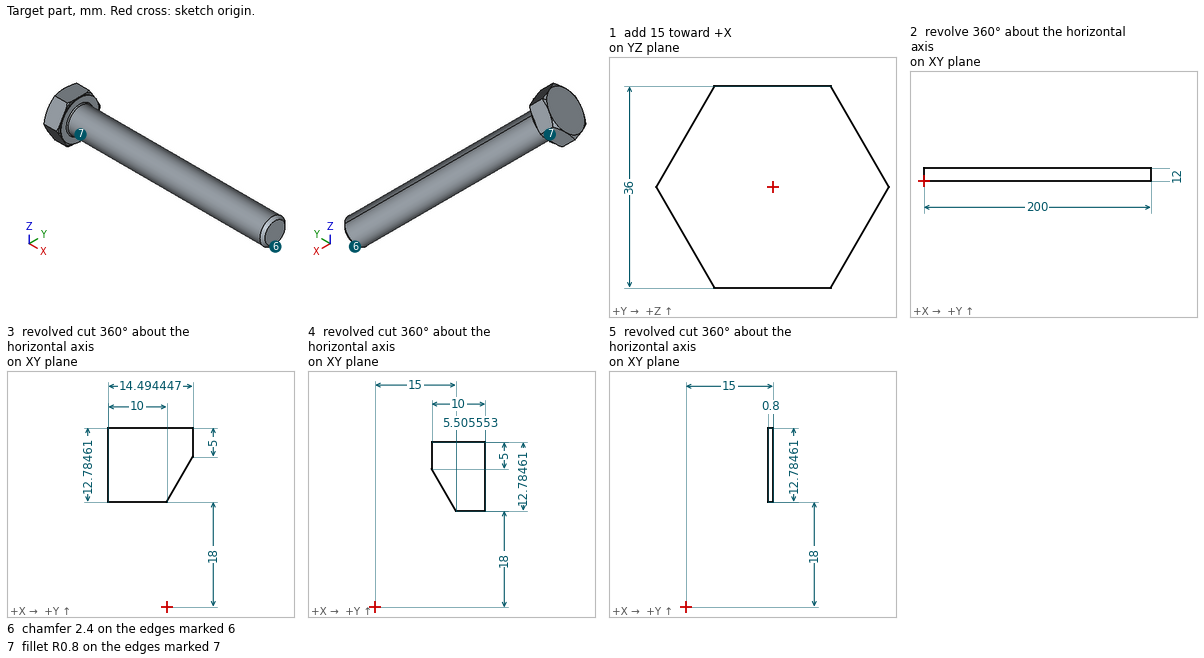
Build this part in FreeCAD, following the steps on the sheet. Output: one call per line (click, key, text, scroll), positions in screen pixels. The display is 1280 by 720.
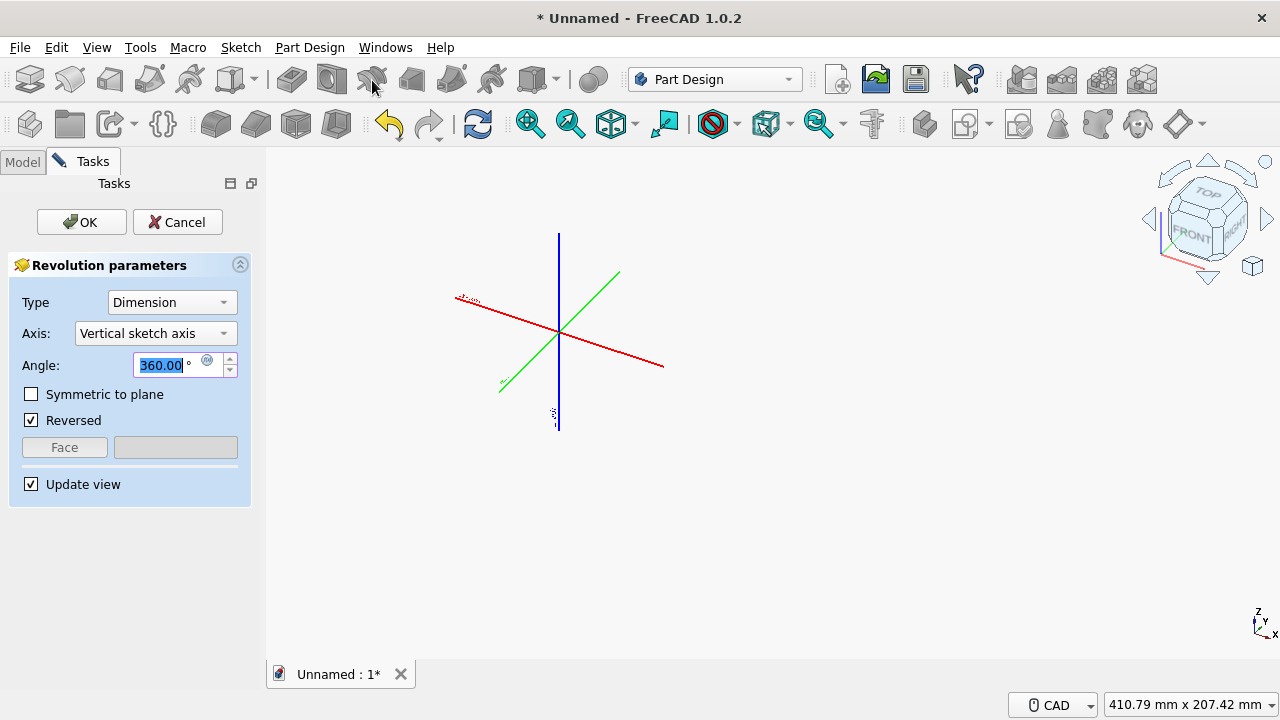
click(156, 334)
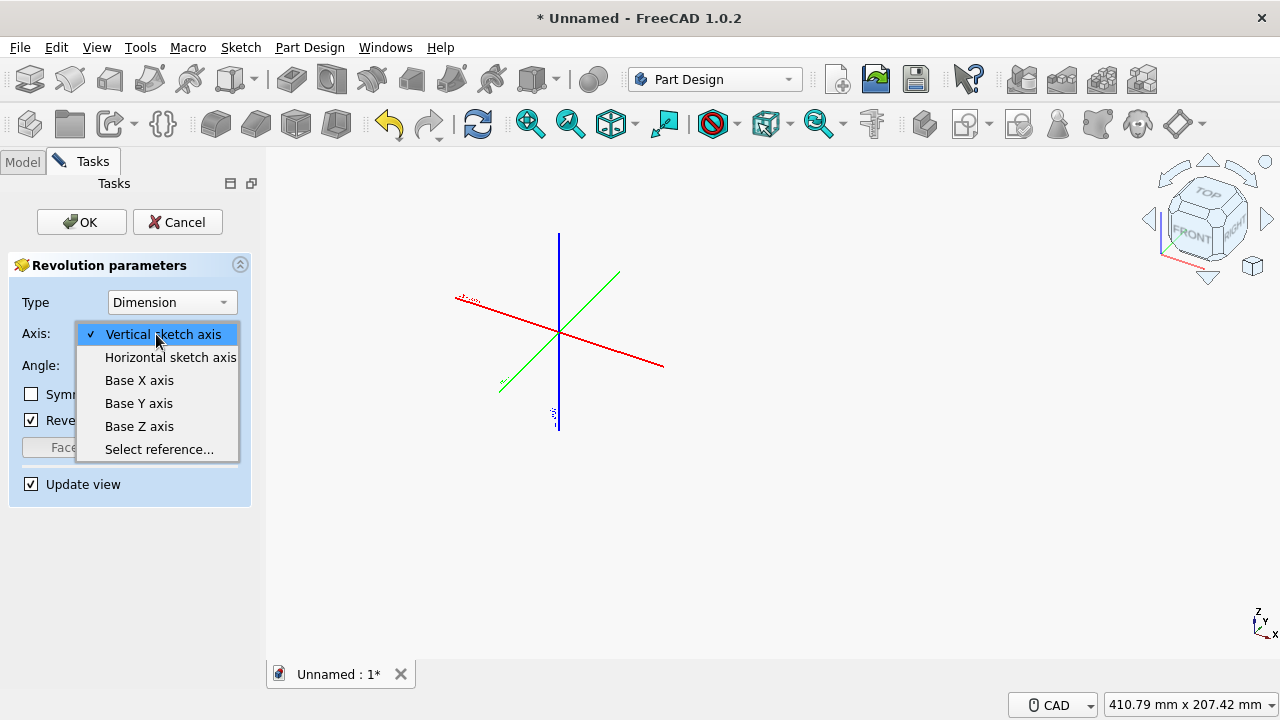
click(156, 358)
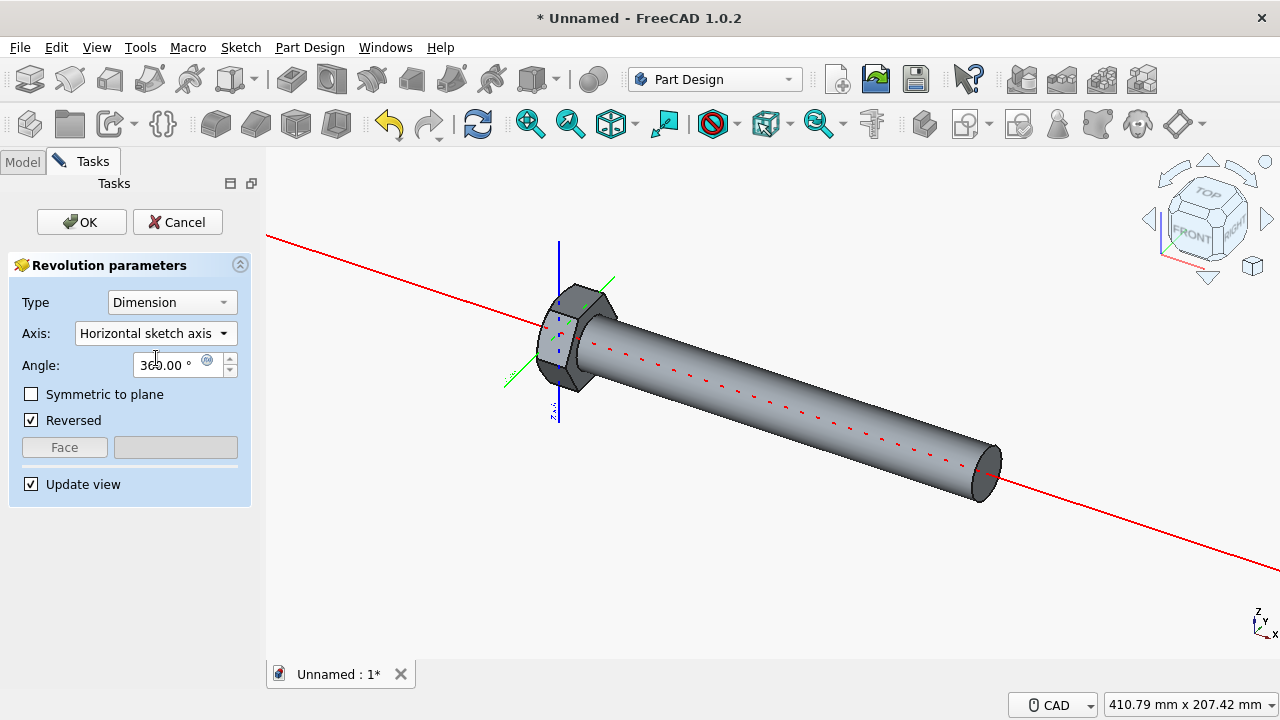
click(82, 222)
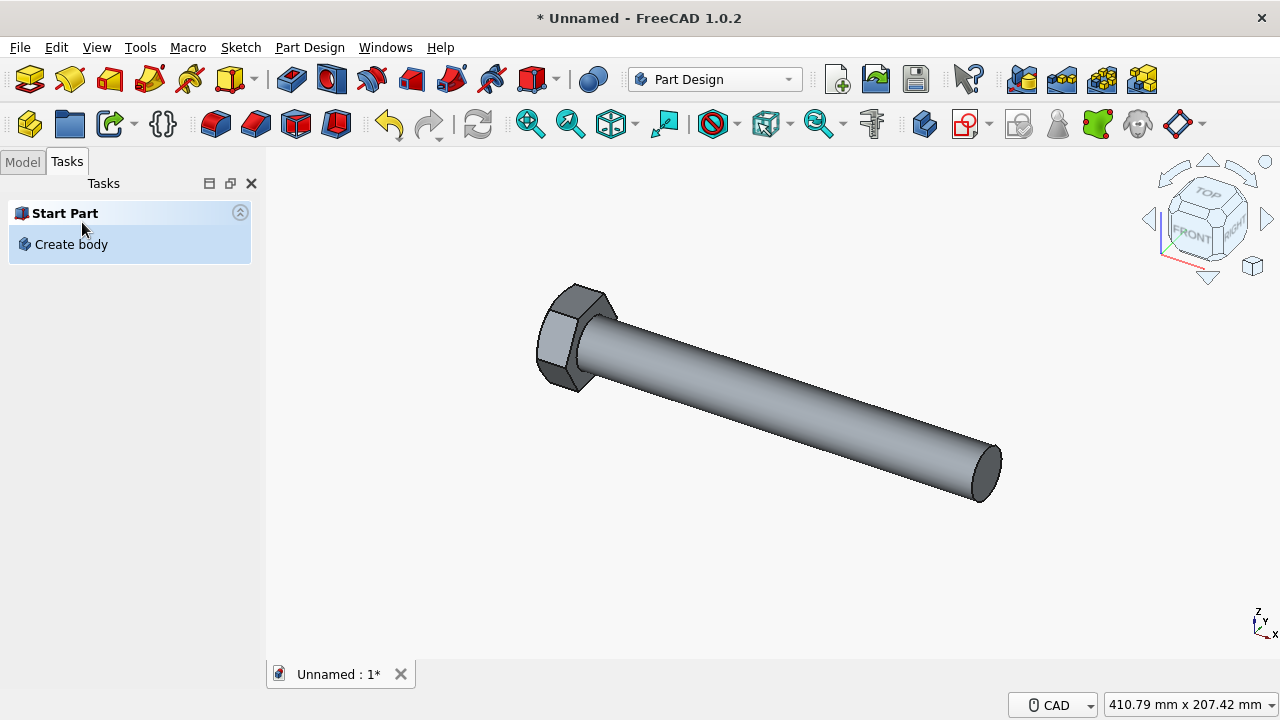
click(966, 124)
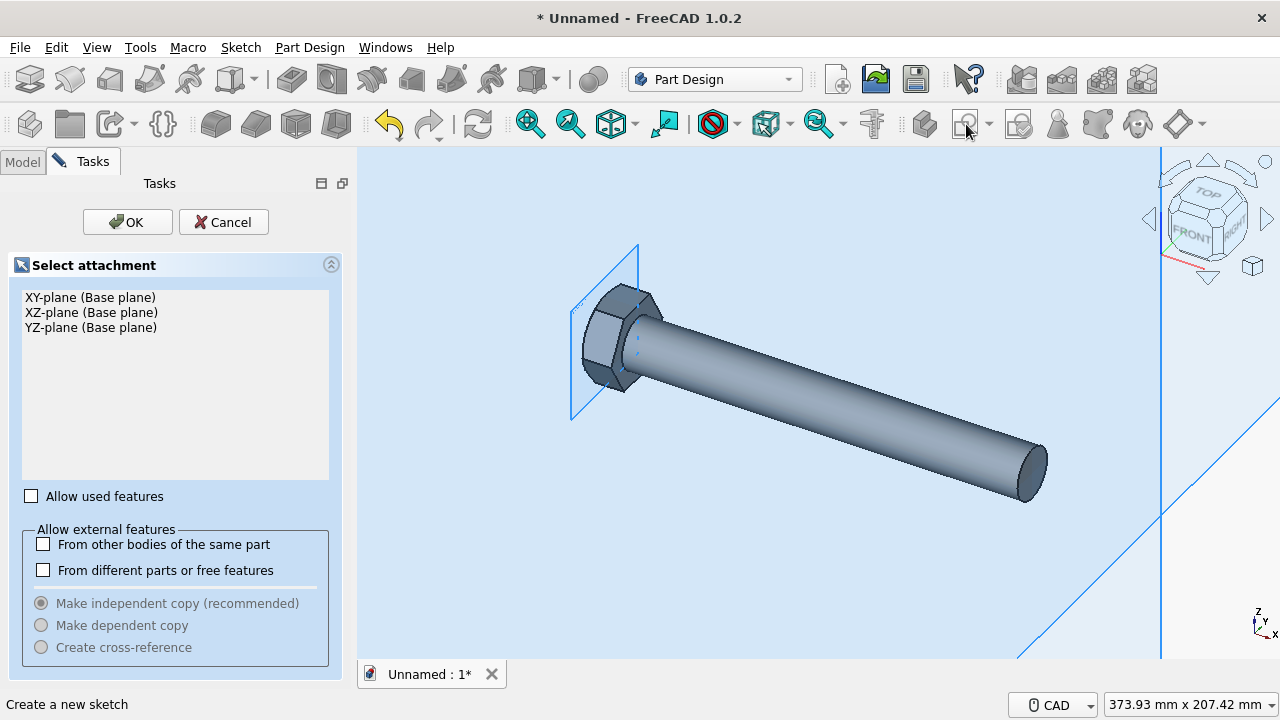
click(82, 298)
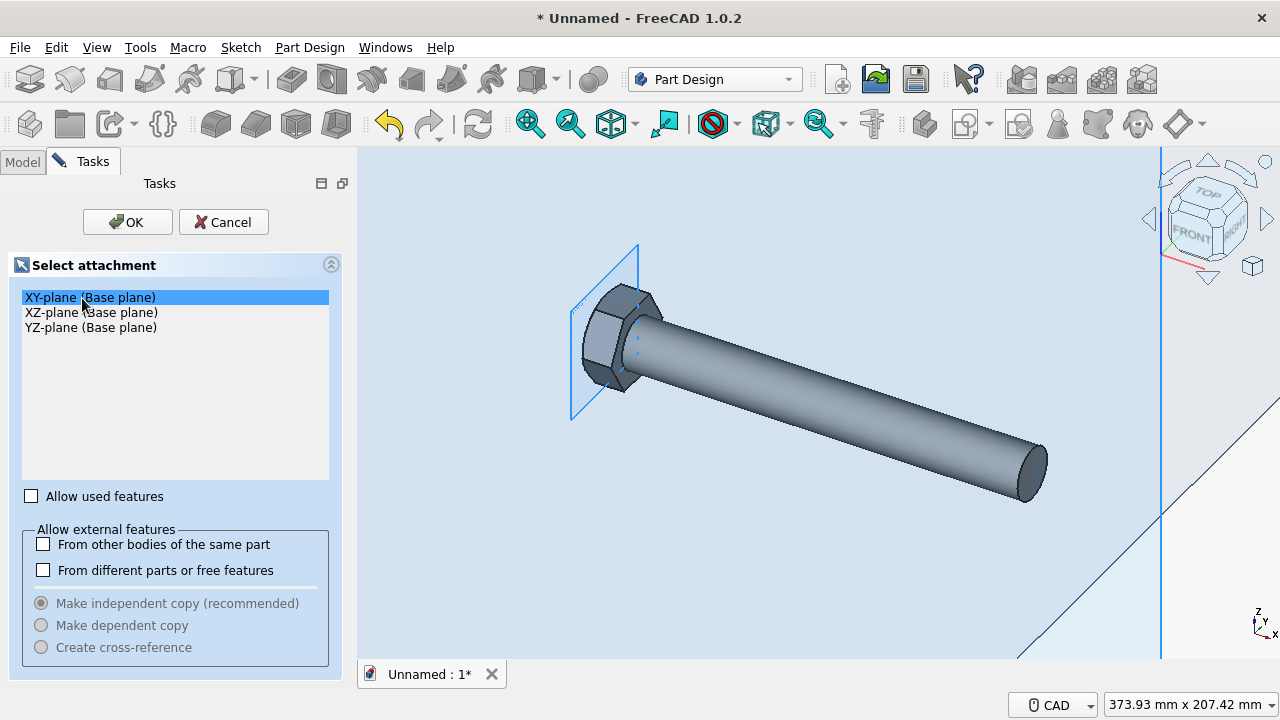
click(128, 222)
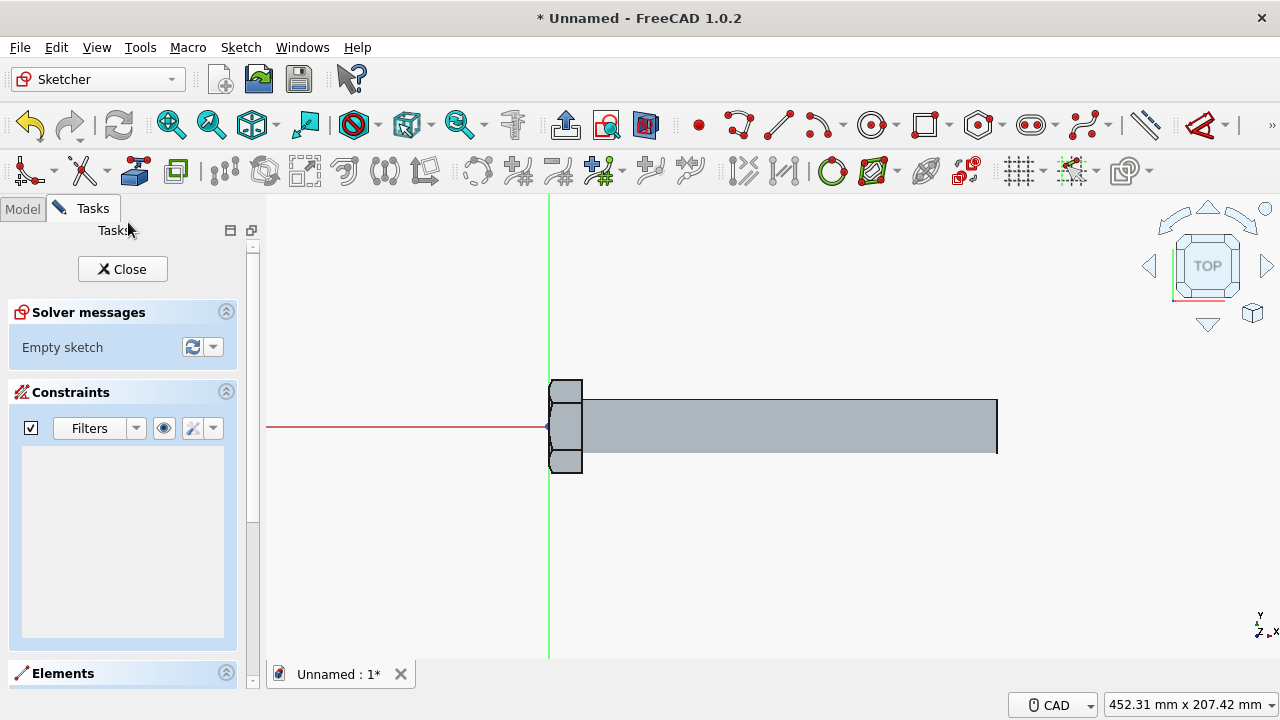
click(646, 126)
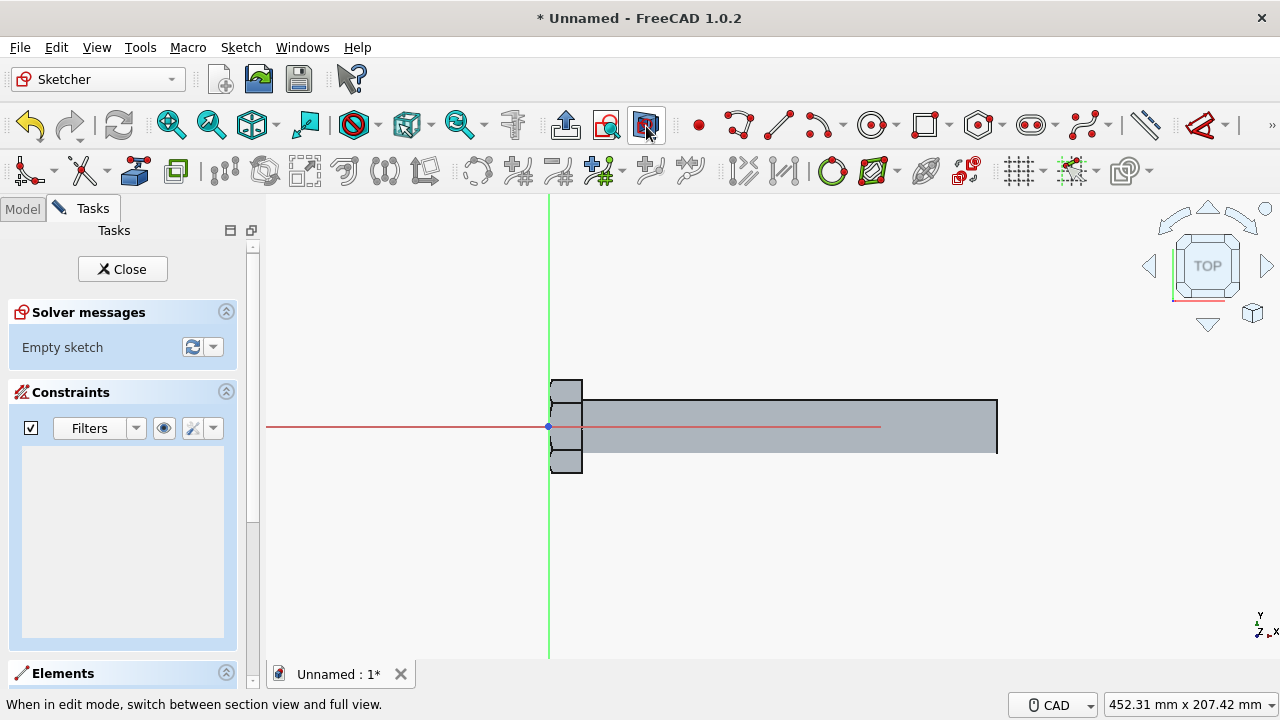
scroll(528, 381, up, 7)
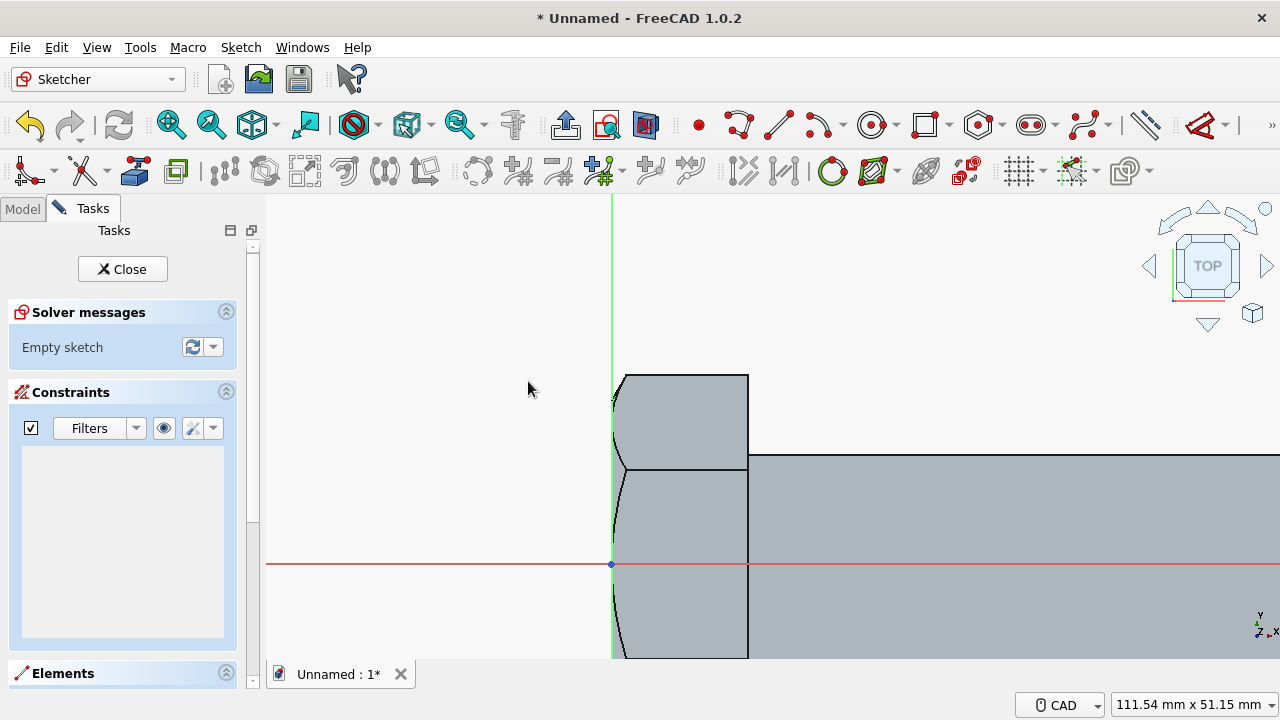
click(740, 126)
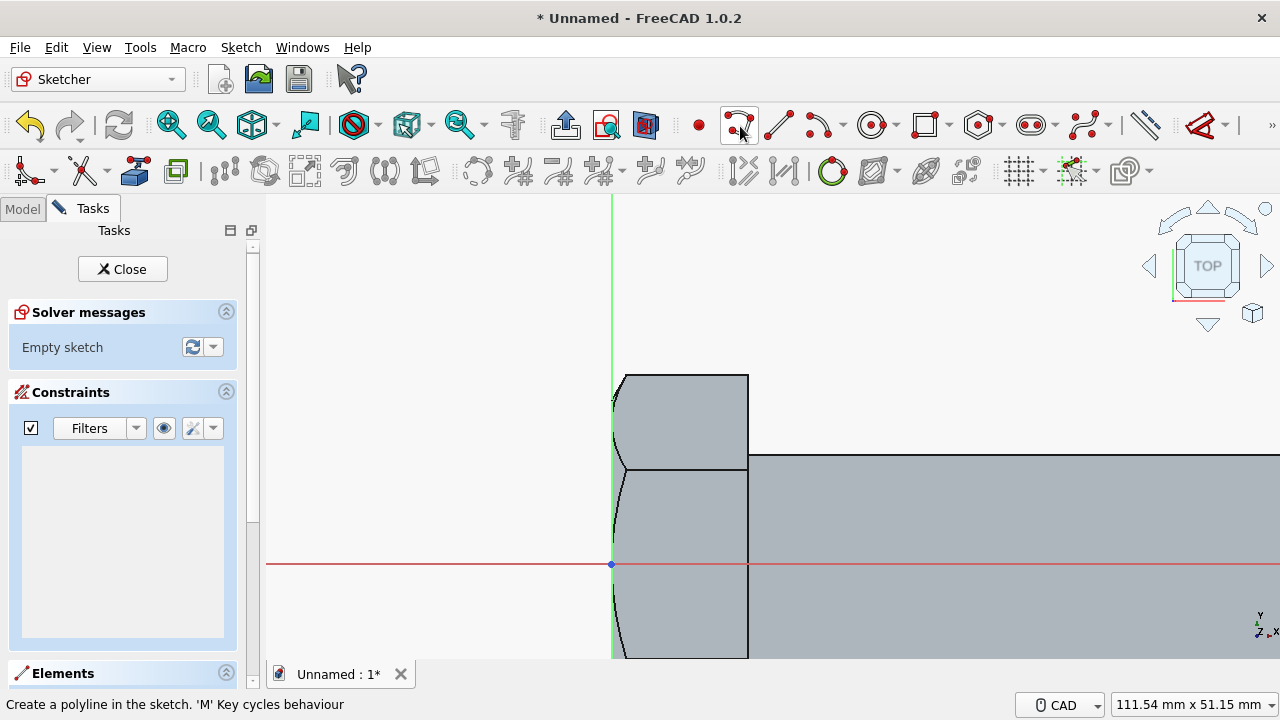
click(748, 401)
click(798, 401)
click(798, 284)
click(707, 284)
click(707, 330)
click(748, 402)
key(Escape)
key(Escape)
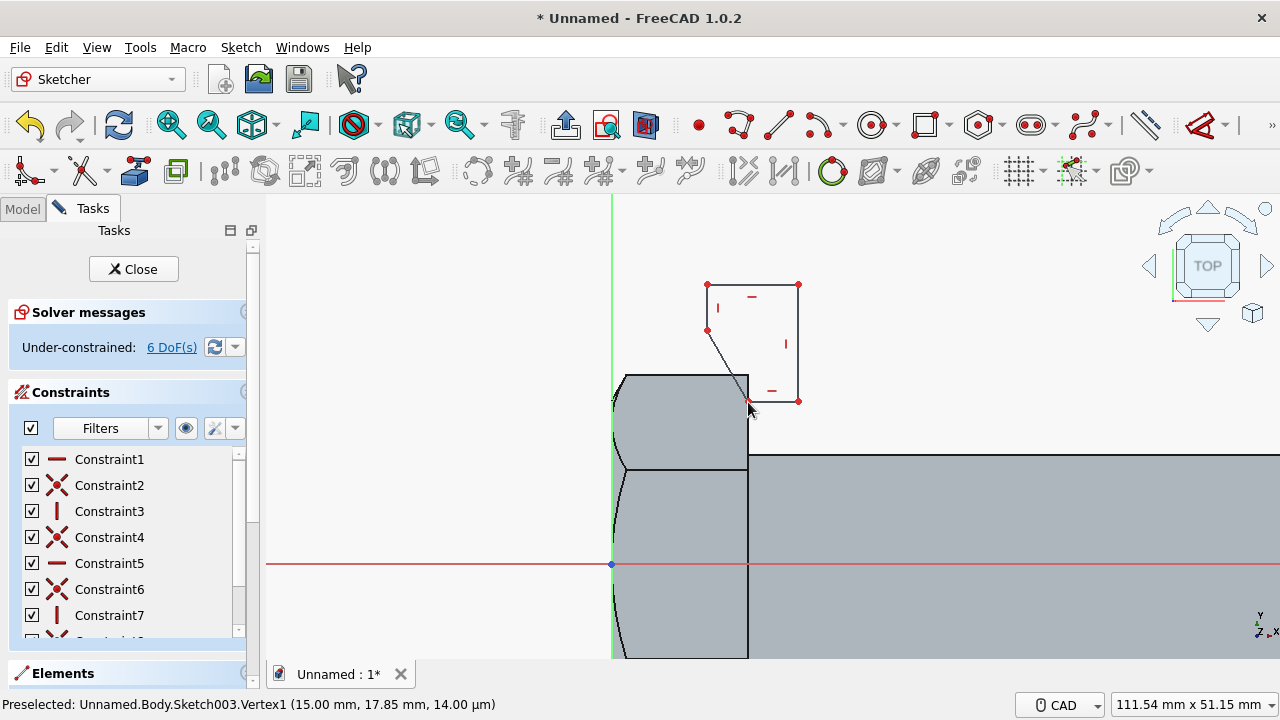
click(1200, 126)